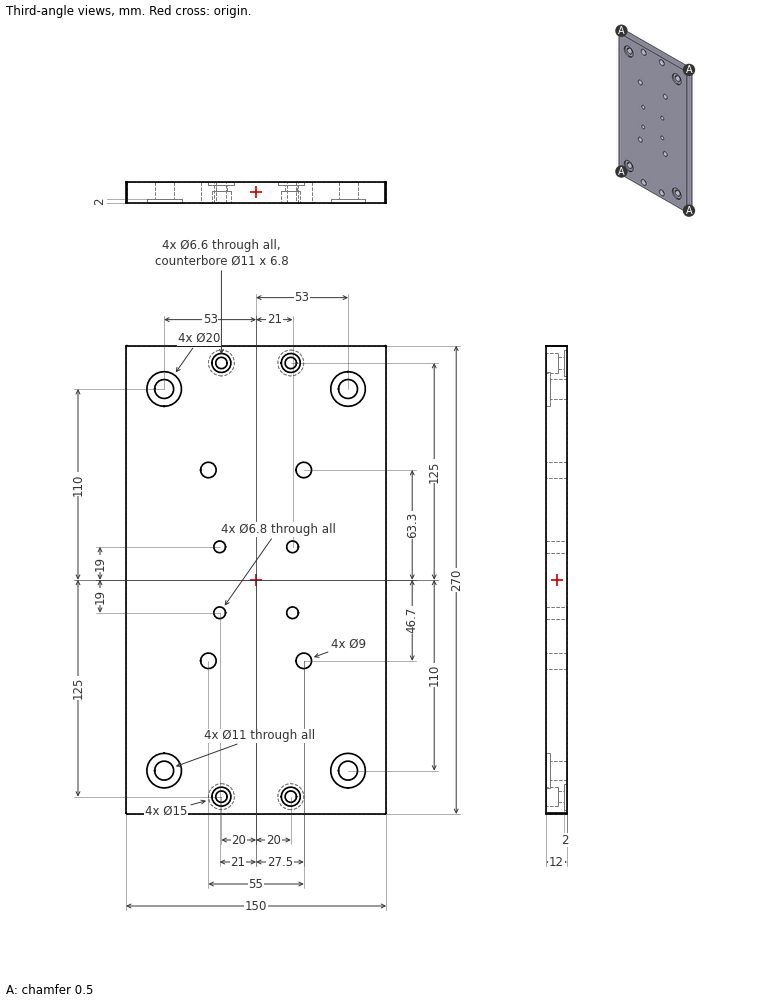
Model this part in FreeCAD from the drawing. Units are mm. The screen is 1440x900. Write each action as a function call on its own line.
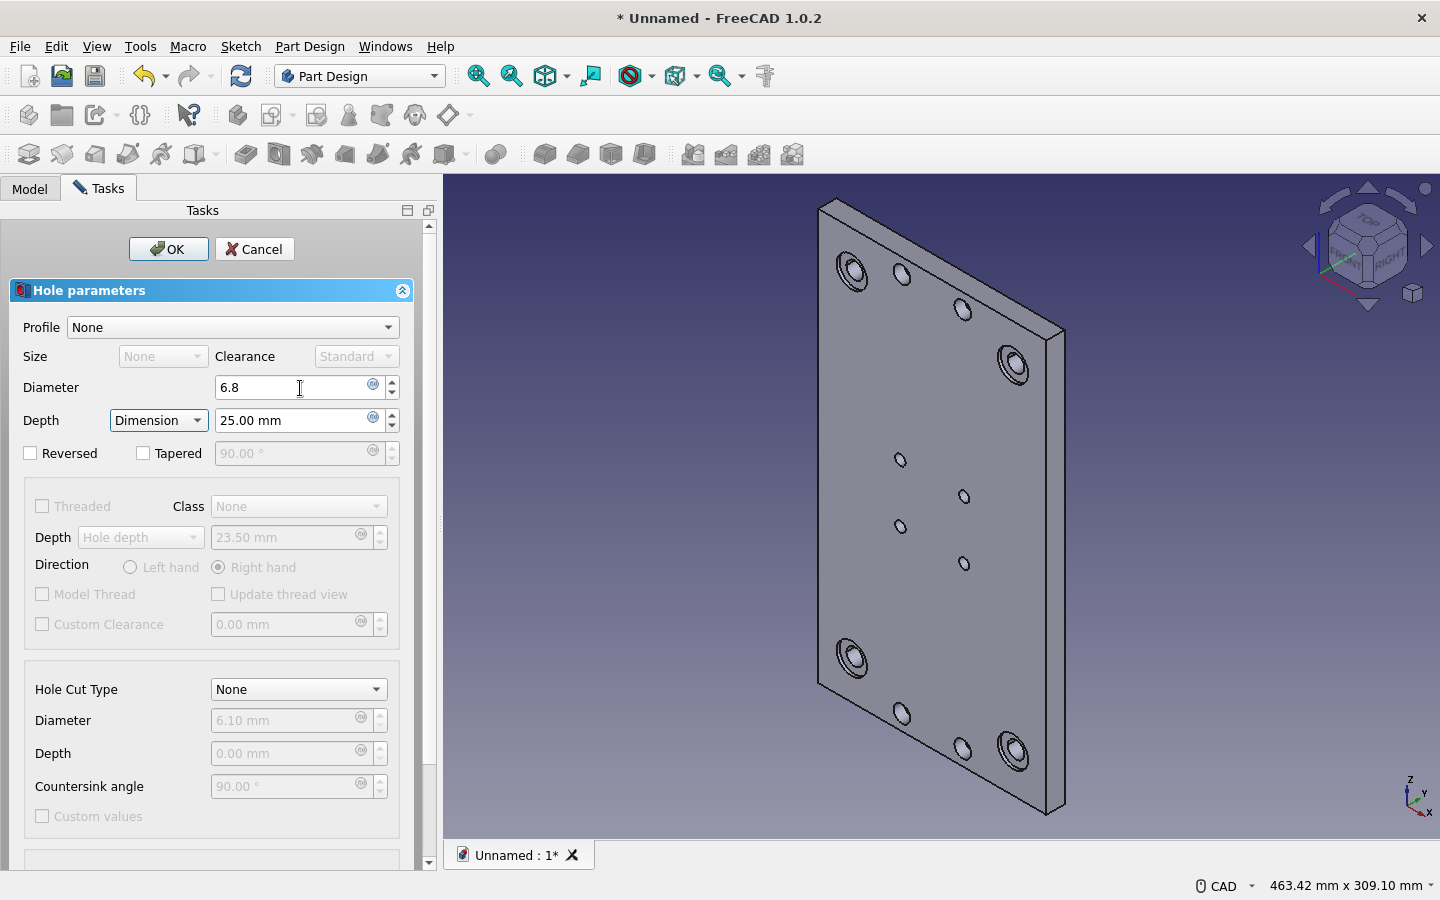
click(160, 420)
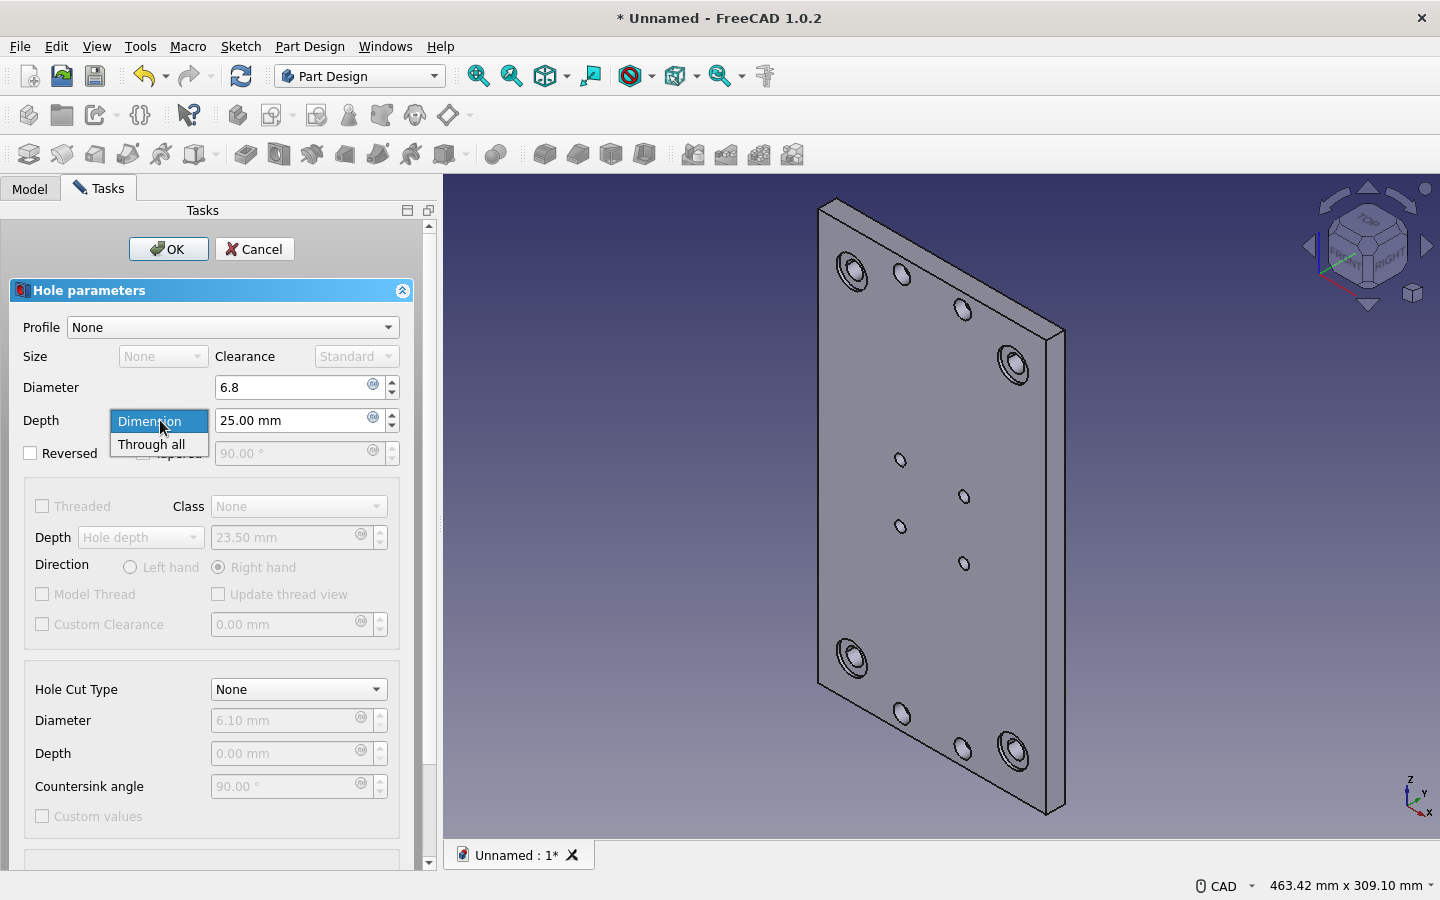
click(158, 444)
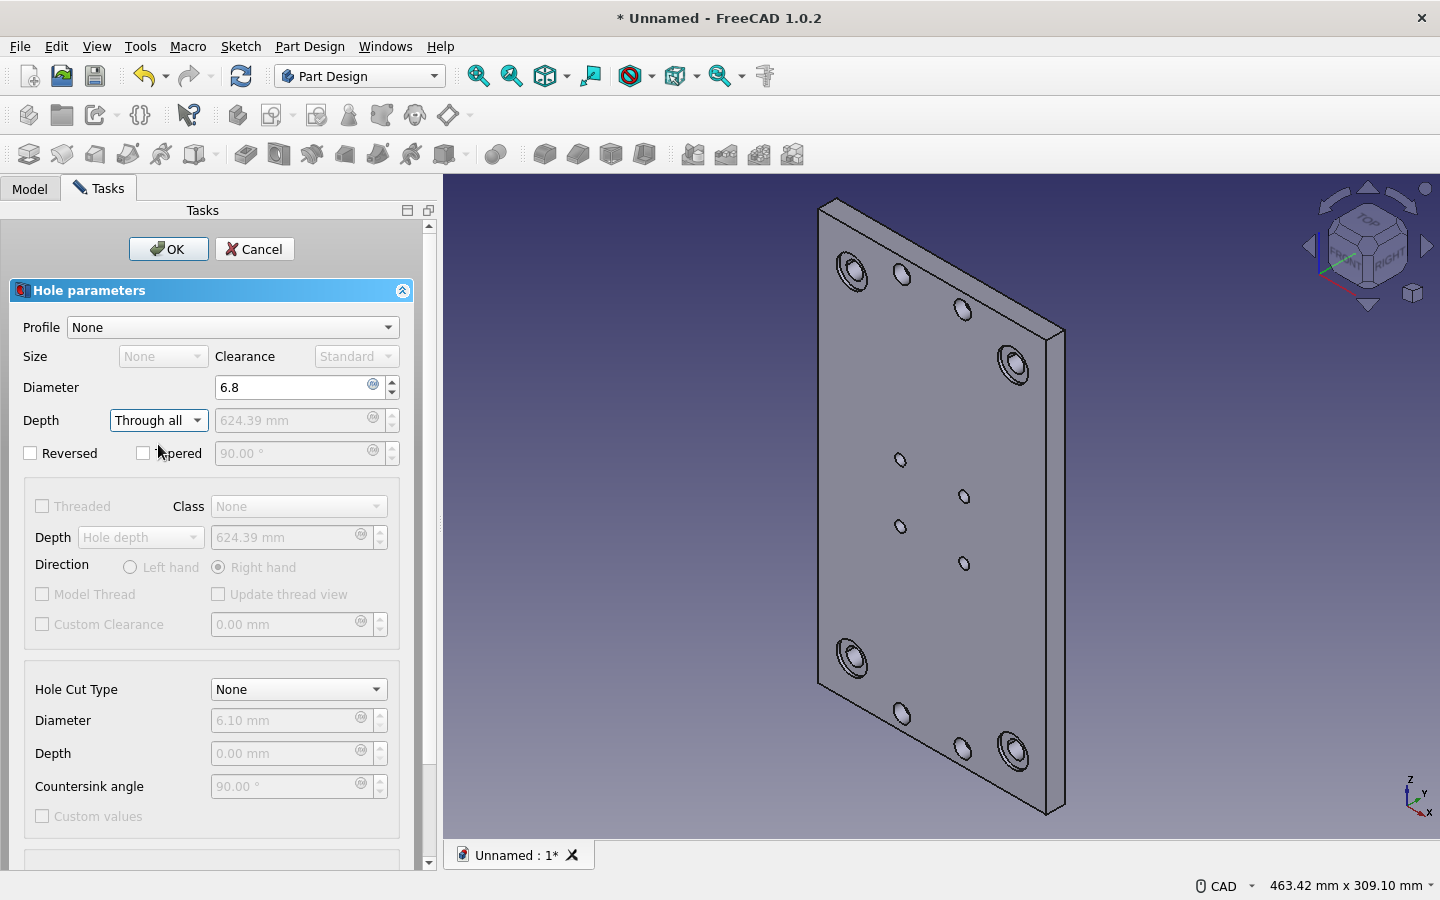
click(169, 249)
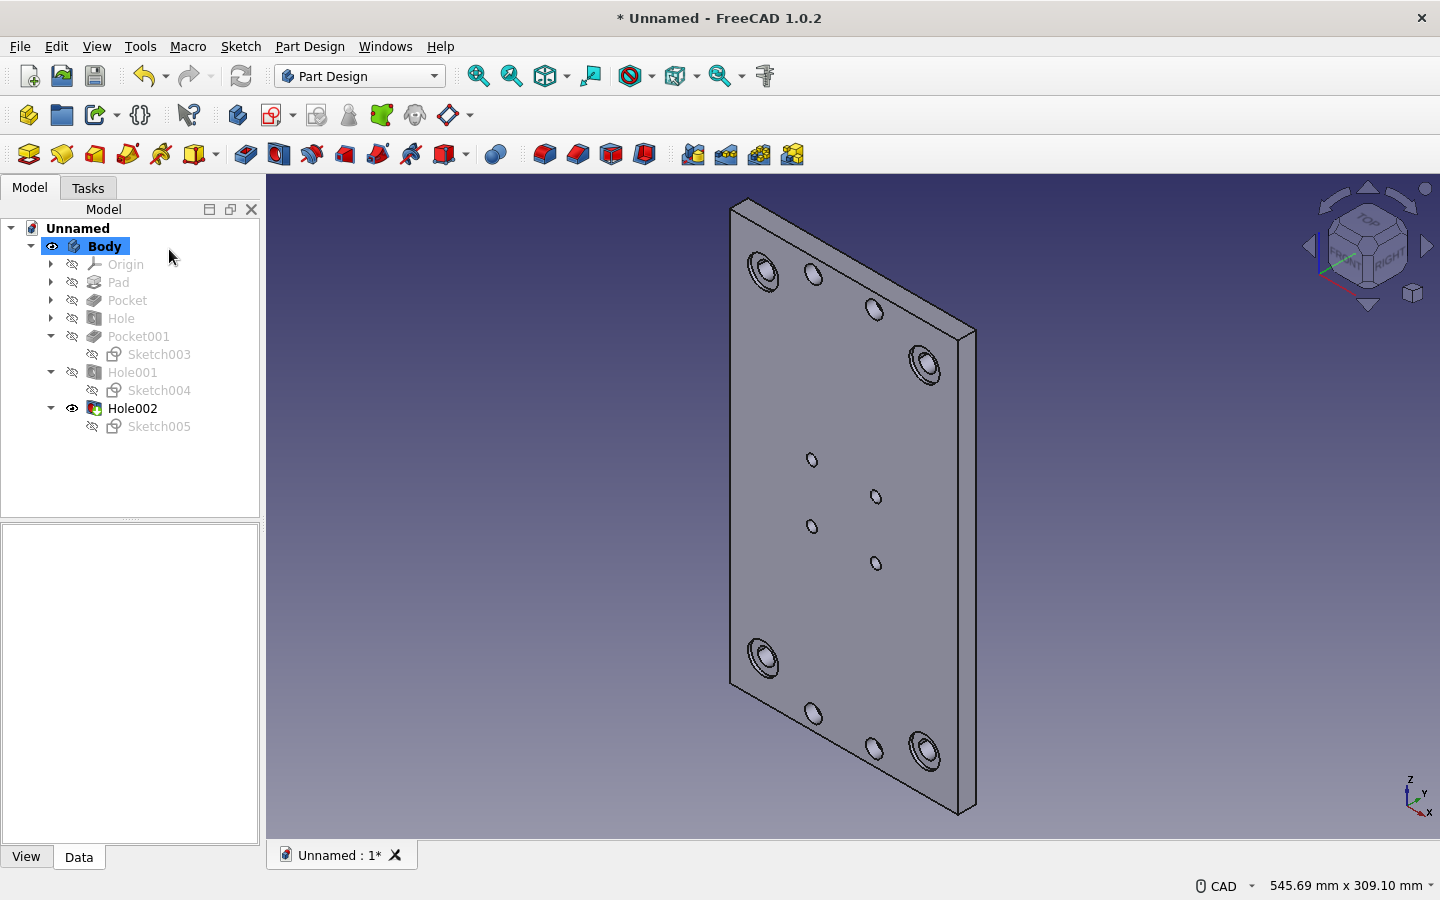
click(967, 334)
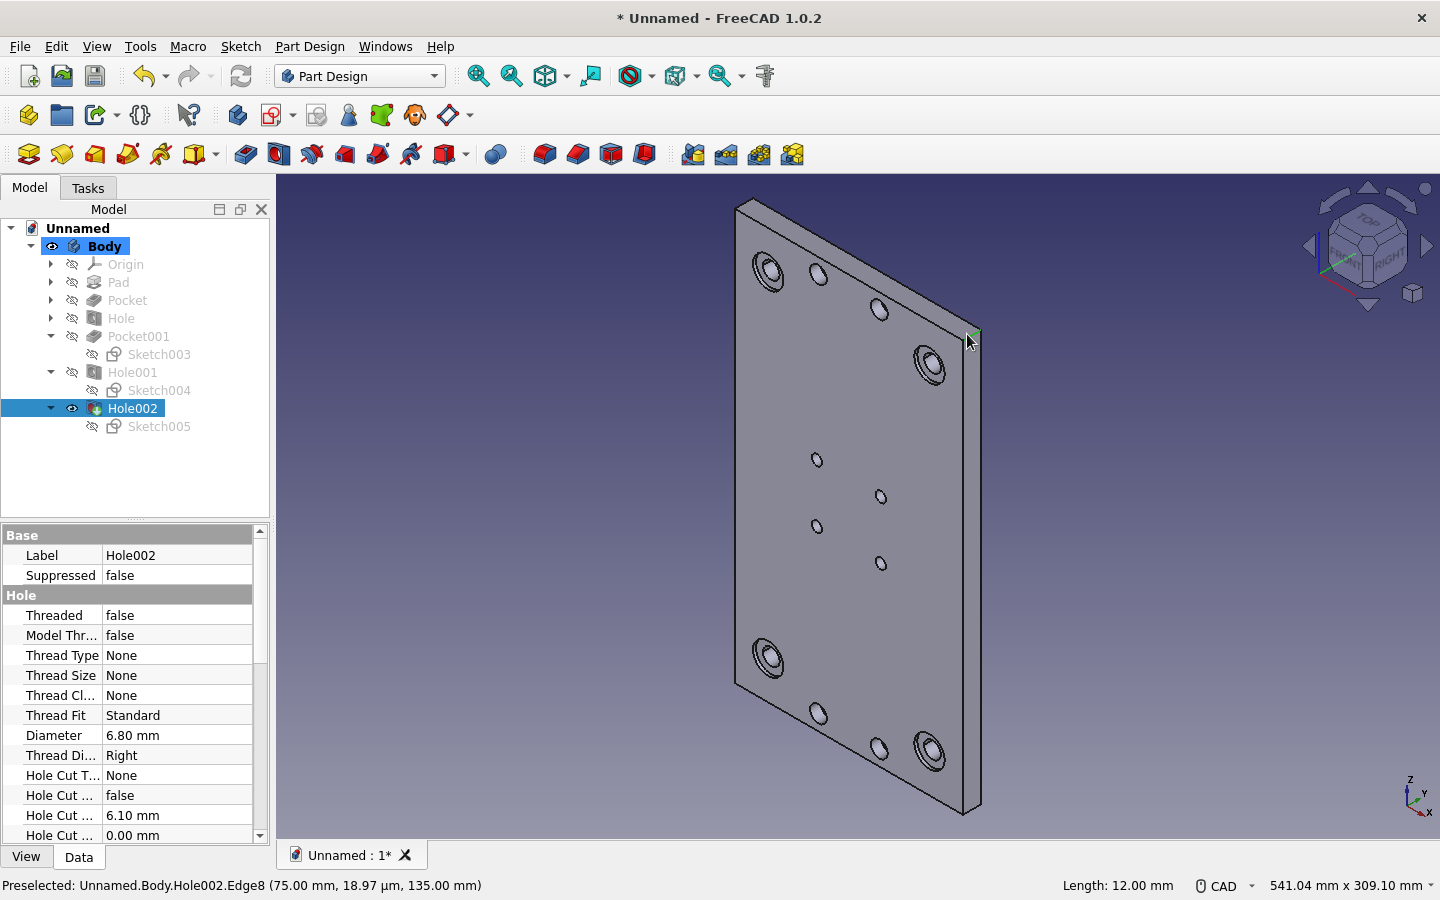
key(2)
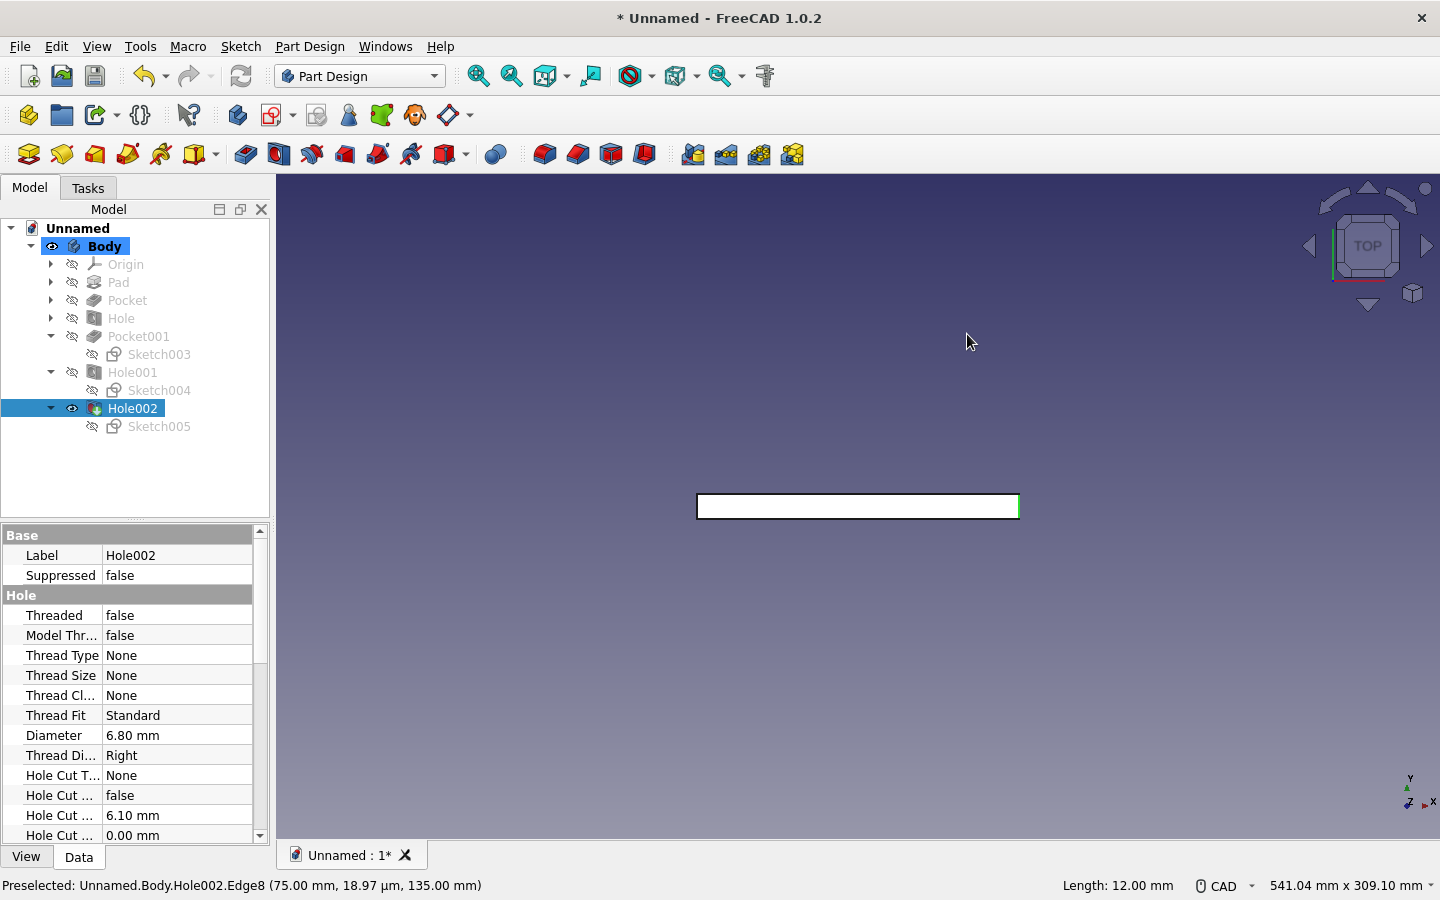
key(v)
key(f)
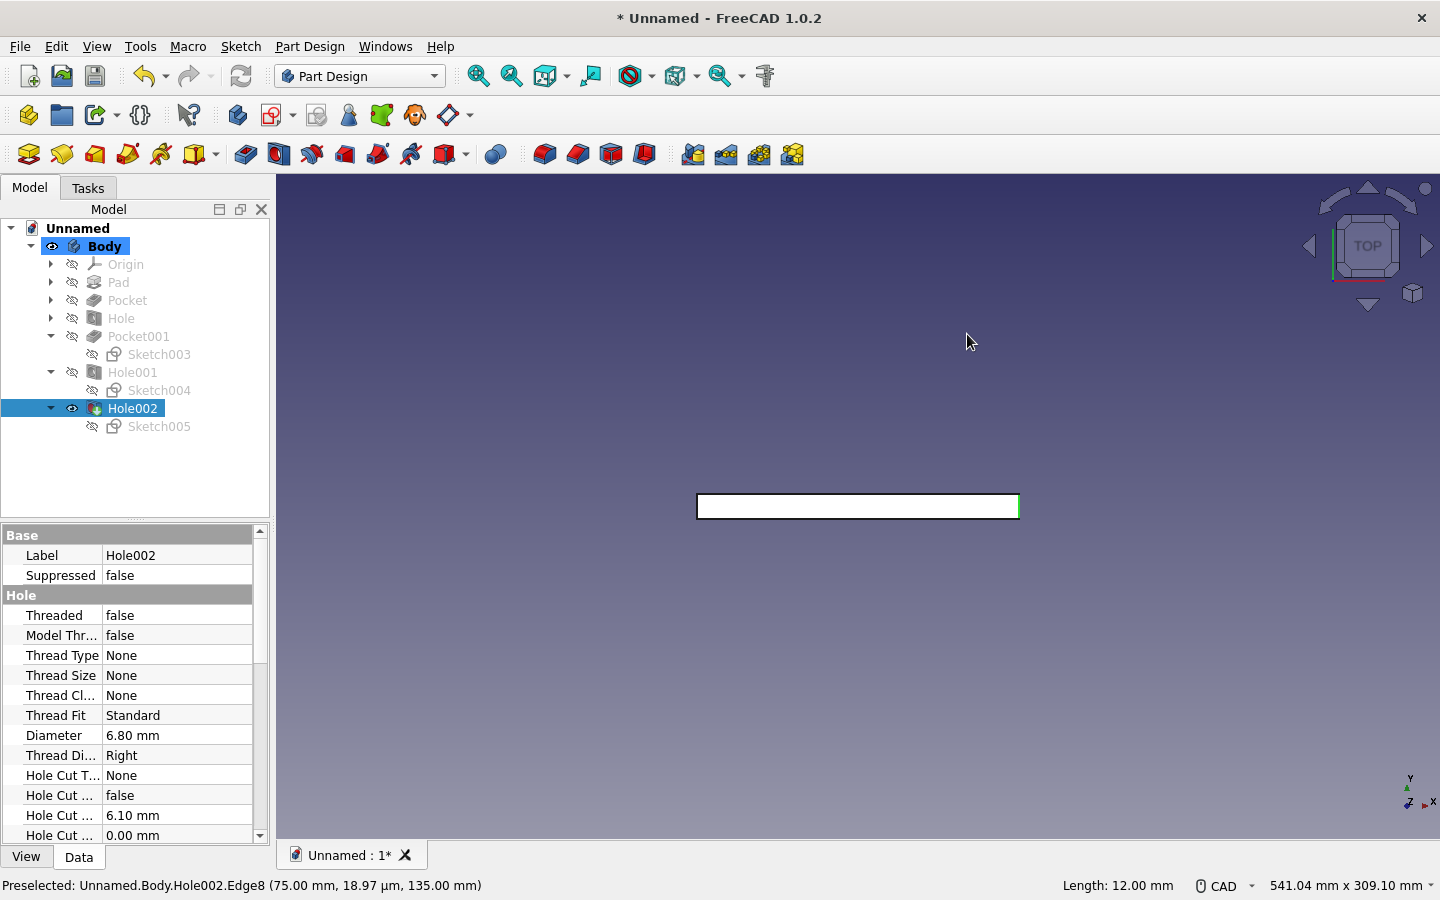
click(697, 505, ctrl)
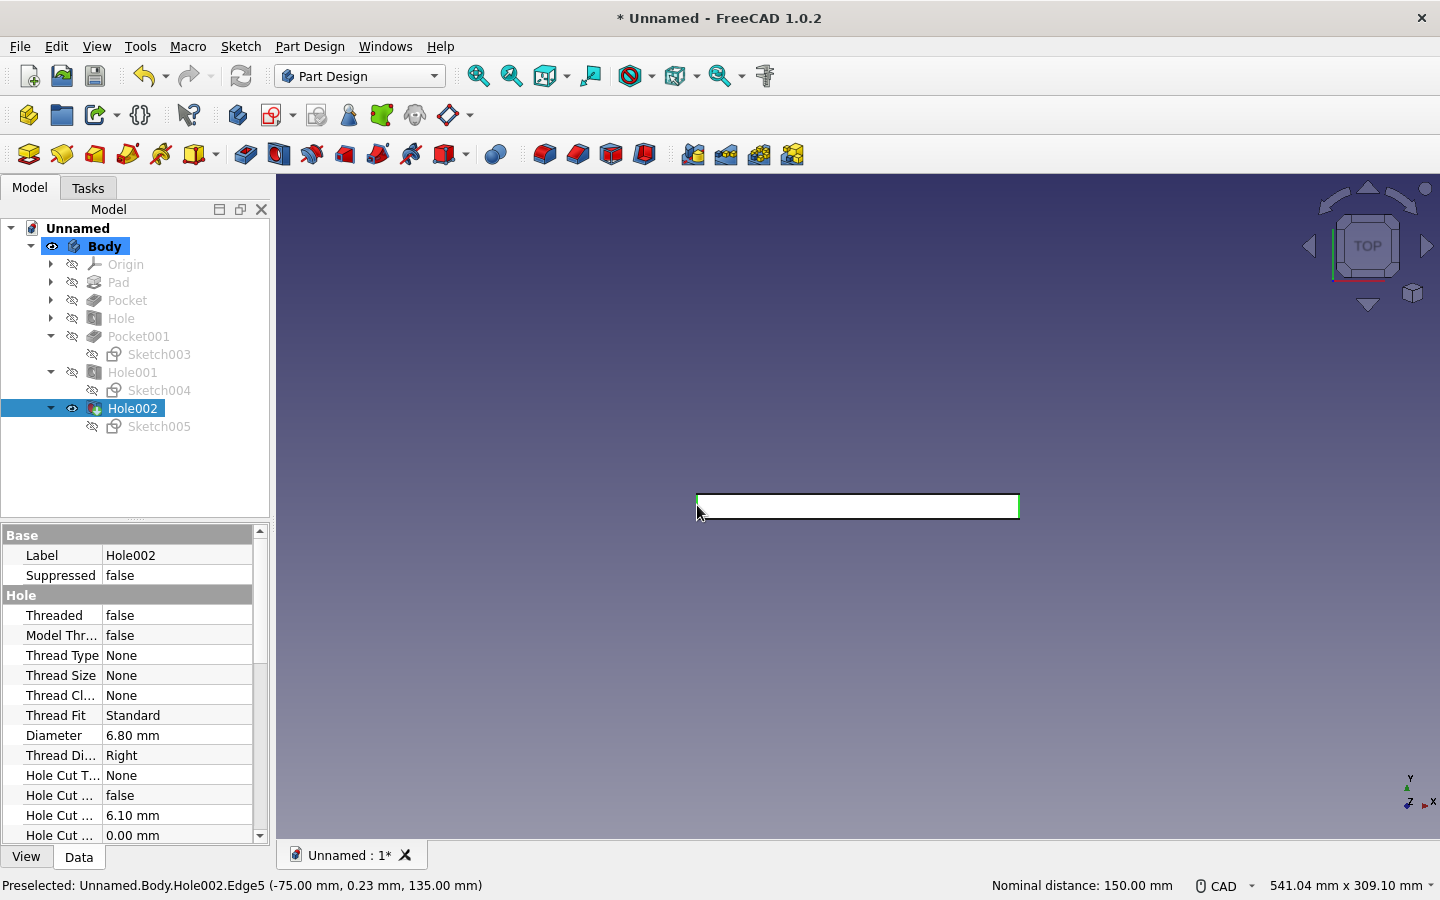
key(0)